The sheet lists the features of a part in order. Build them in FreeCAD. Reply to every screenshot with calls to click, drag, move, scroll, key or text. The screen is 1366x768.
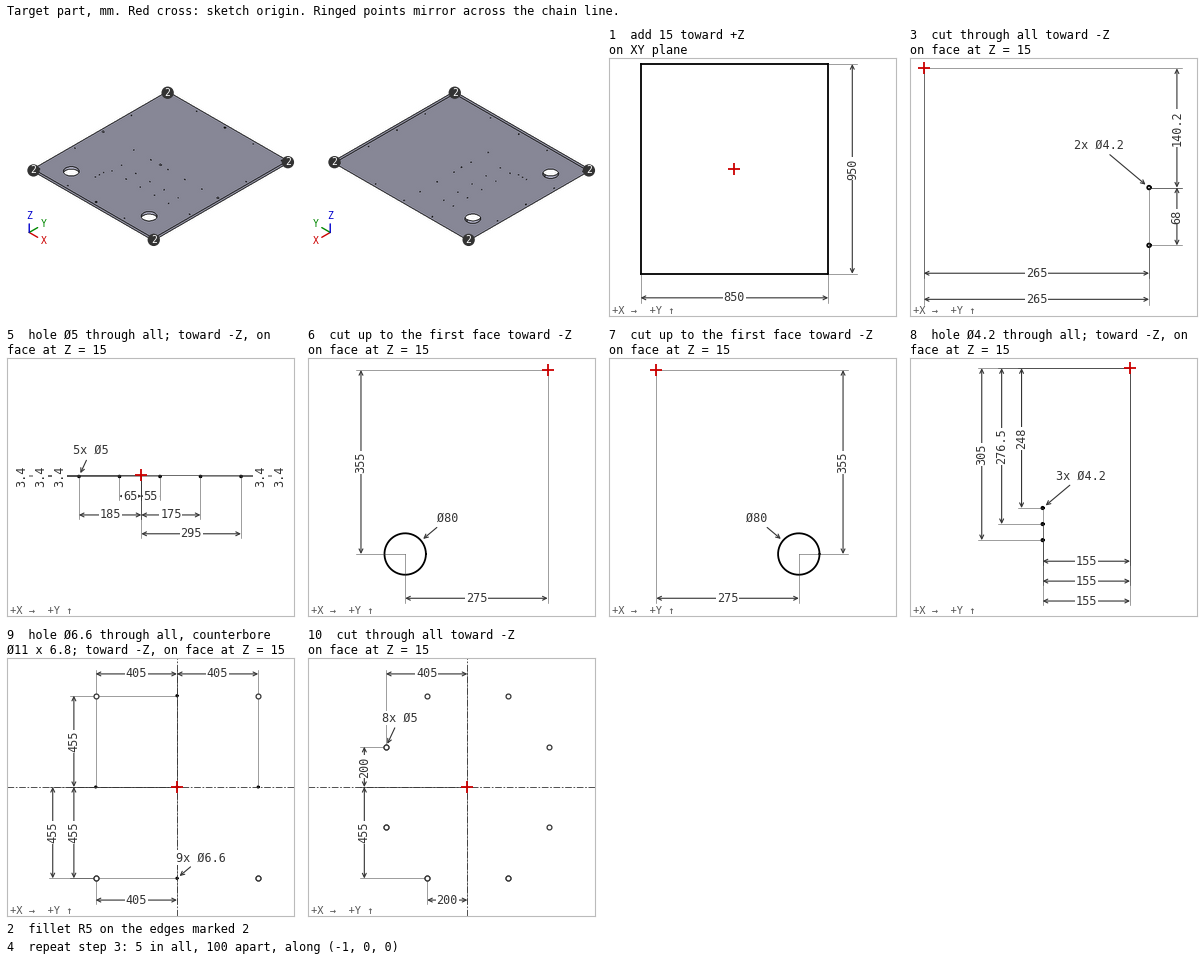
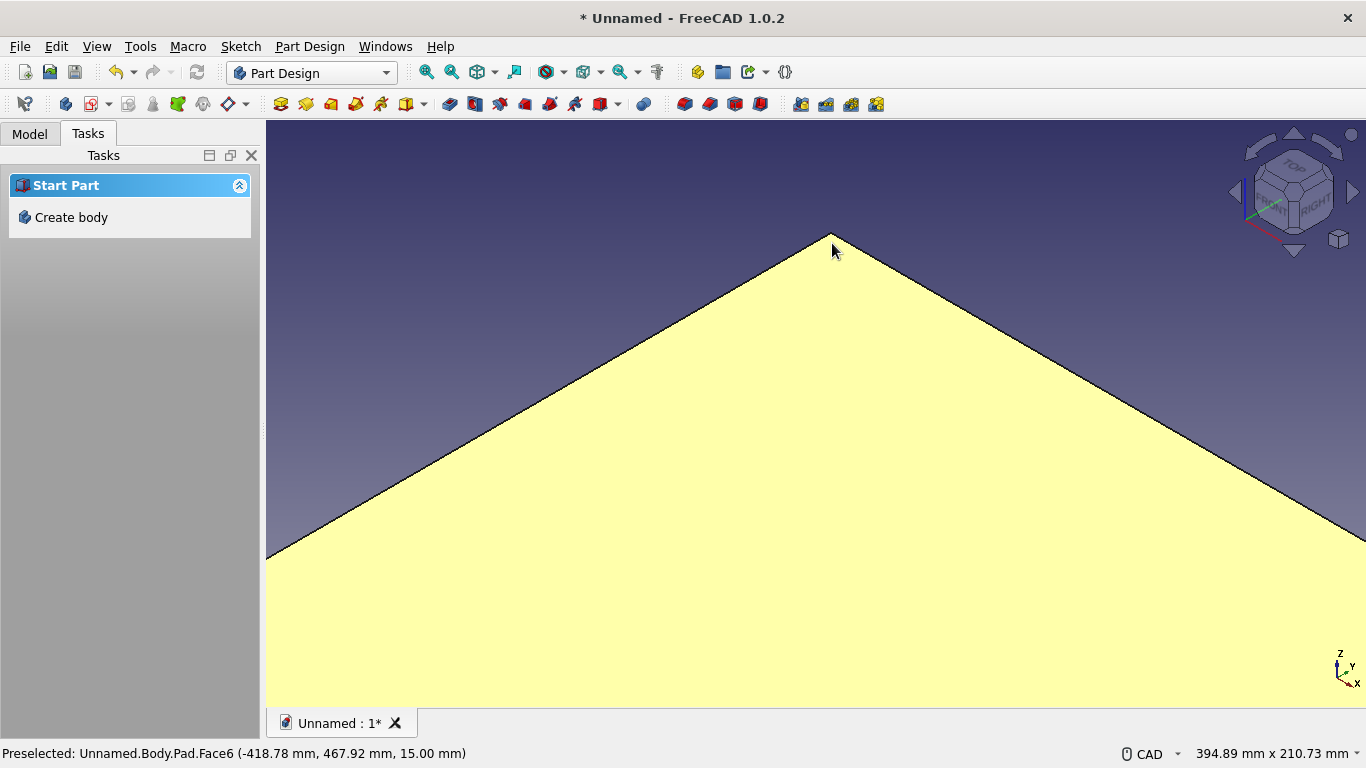
click(427, 72)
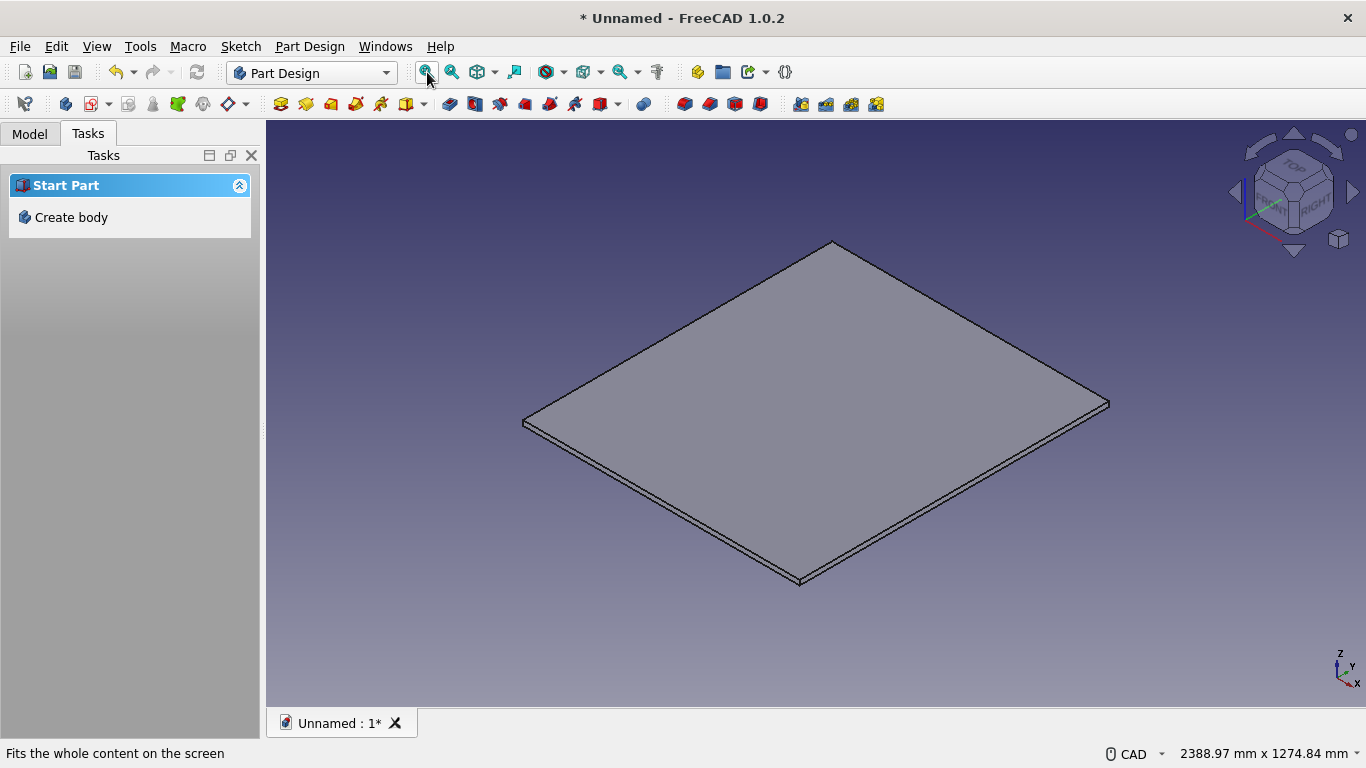
key(2)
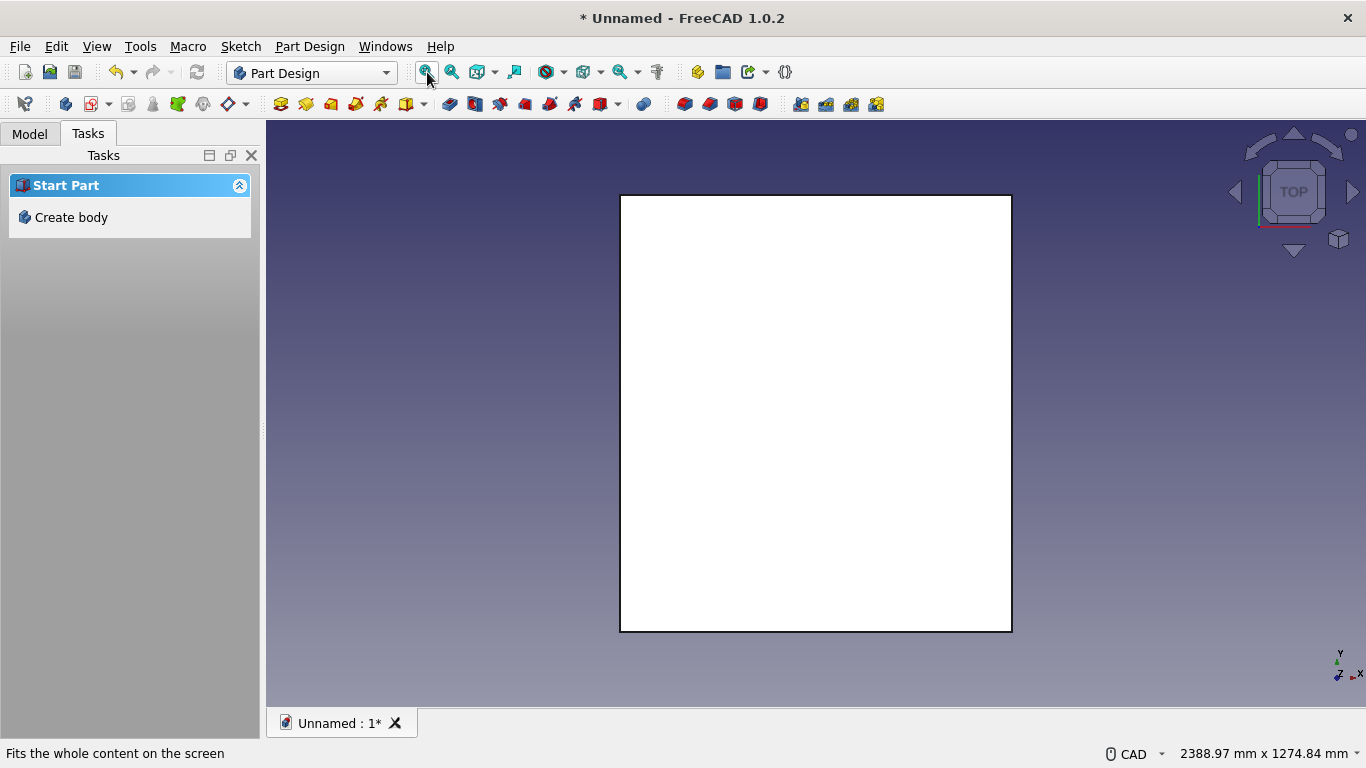
scroll(620, 194, up, 9)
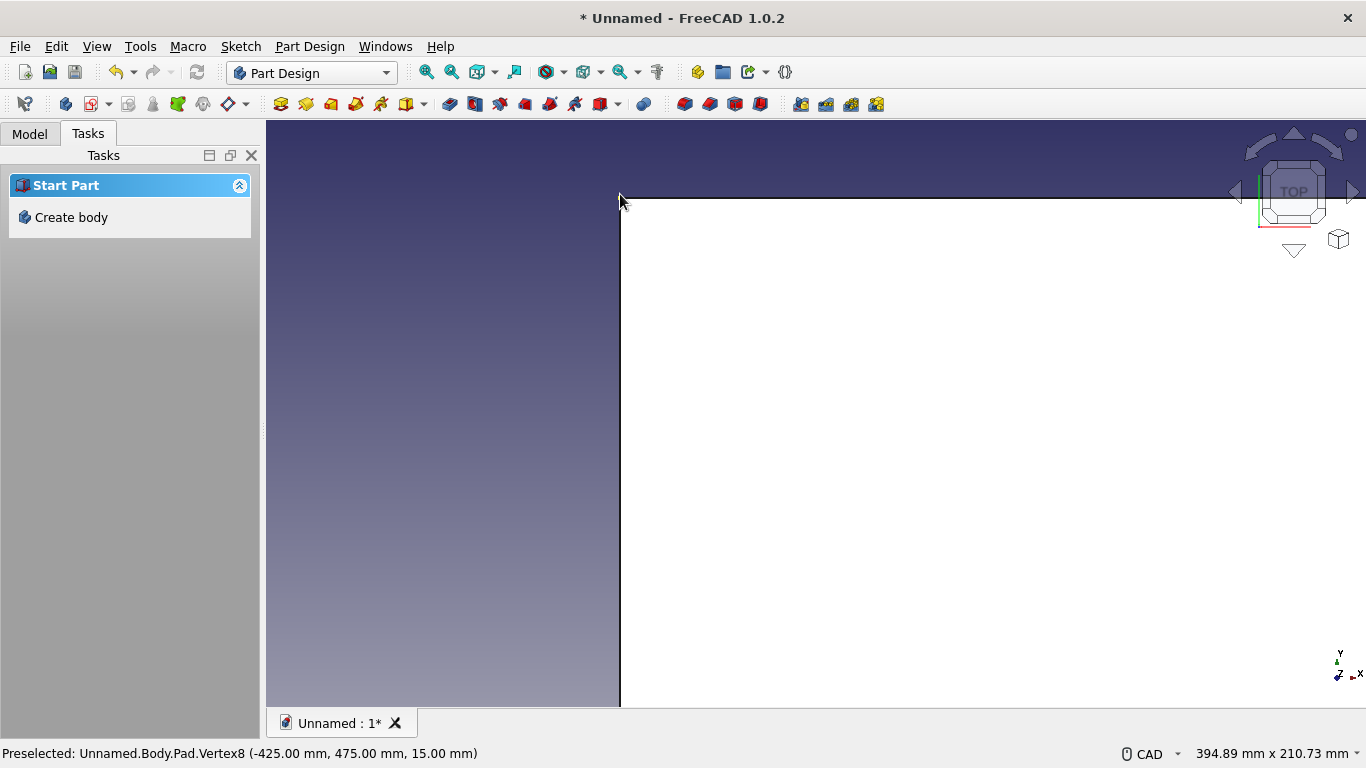
click(427, 72)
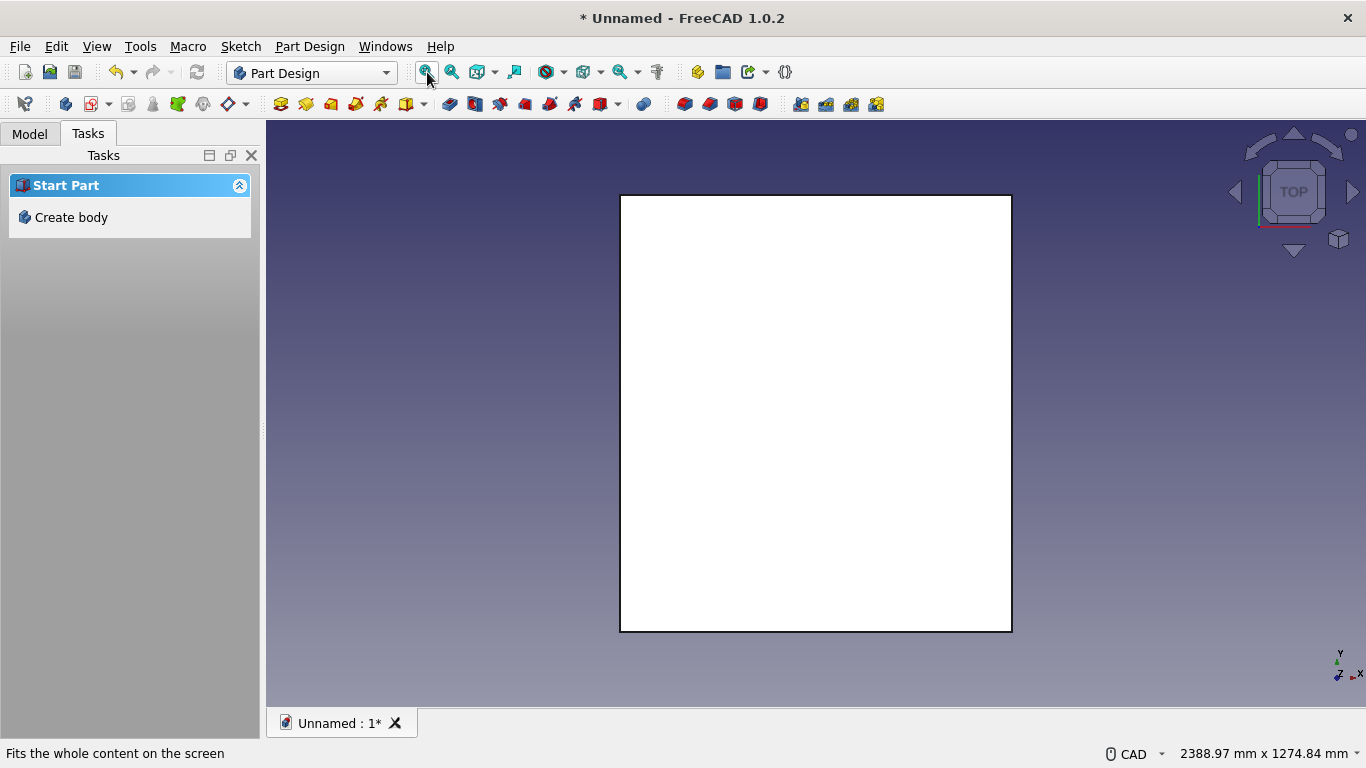
key(1)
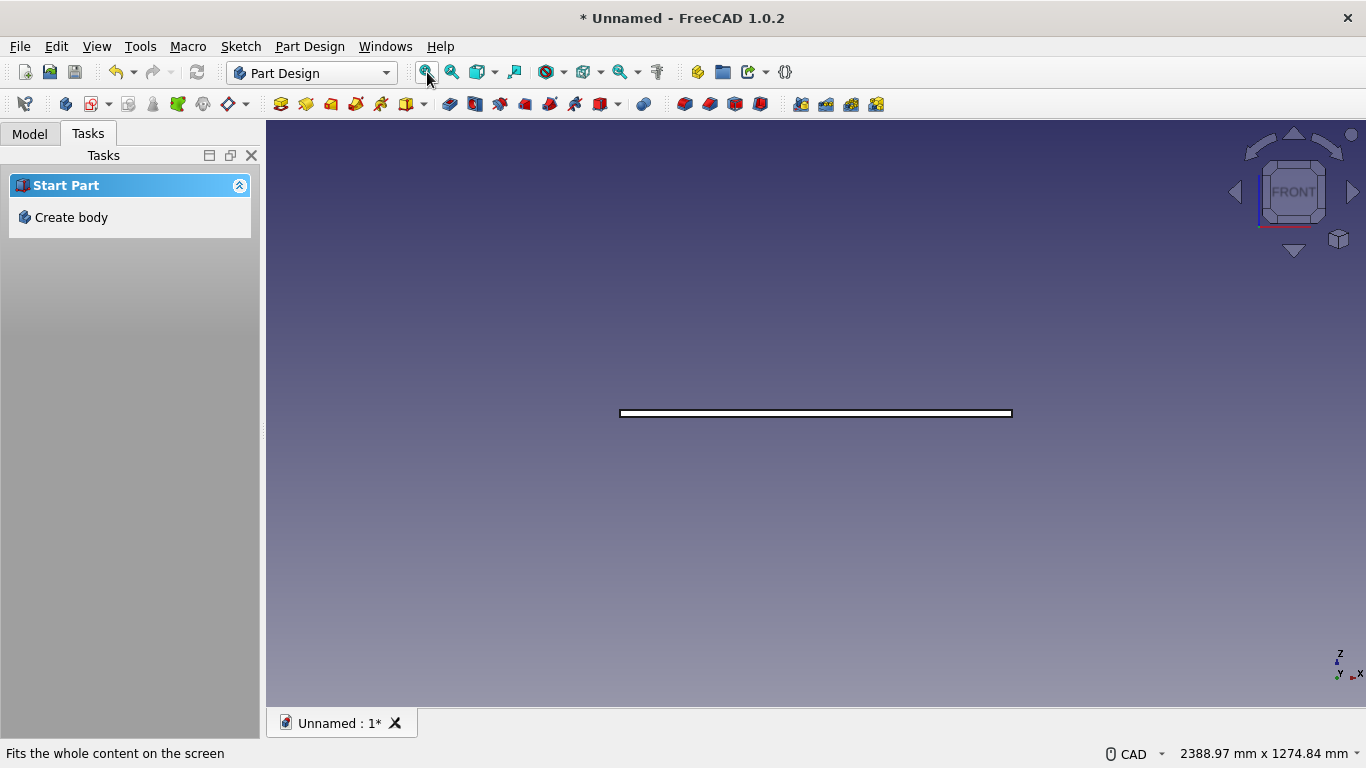
click(427, 72)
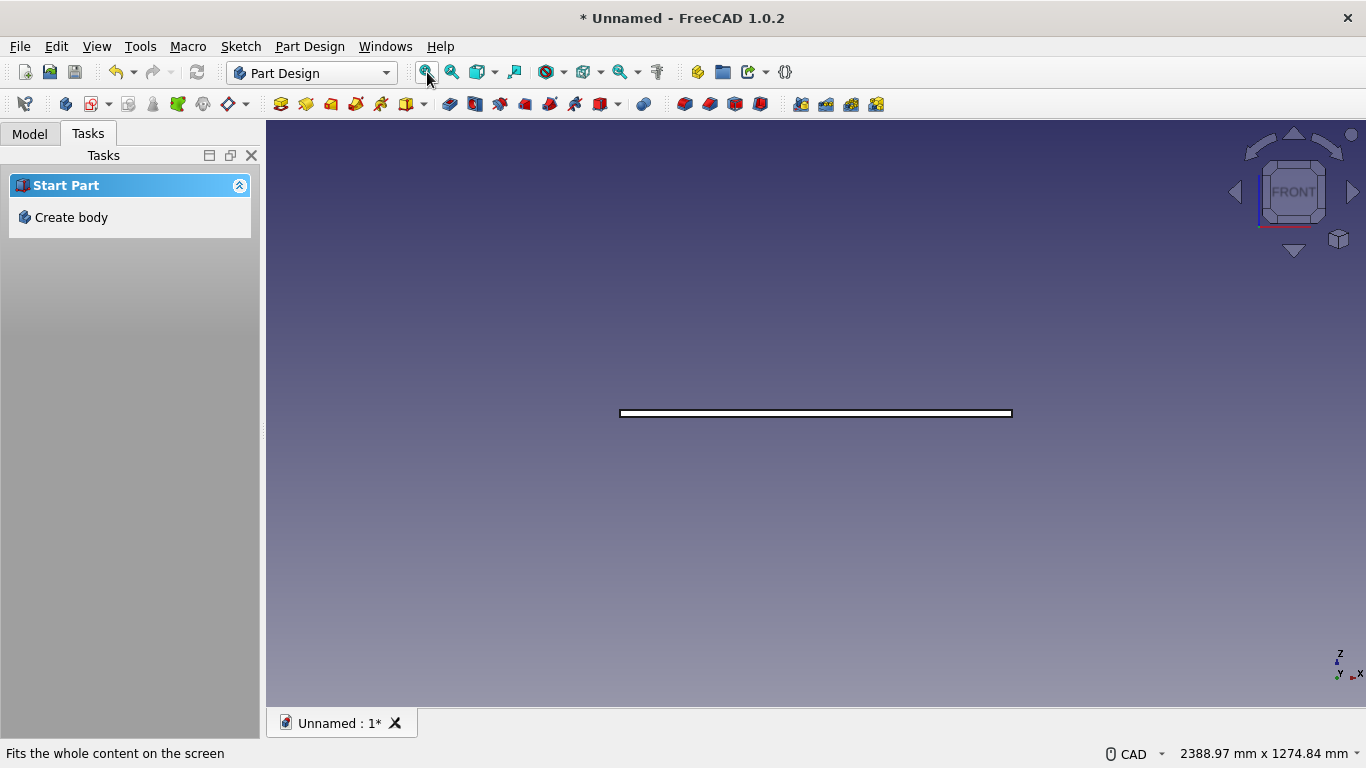
scroll(620, 413, up, 9)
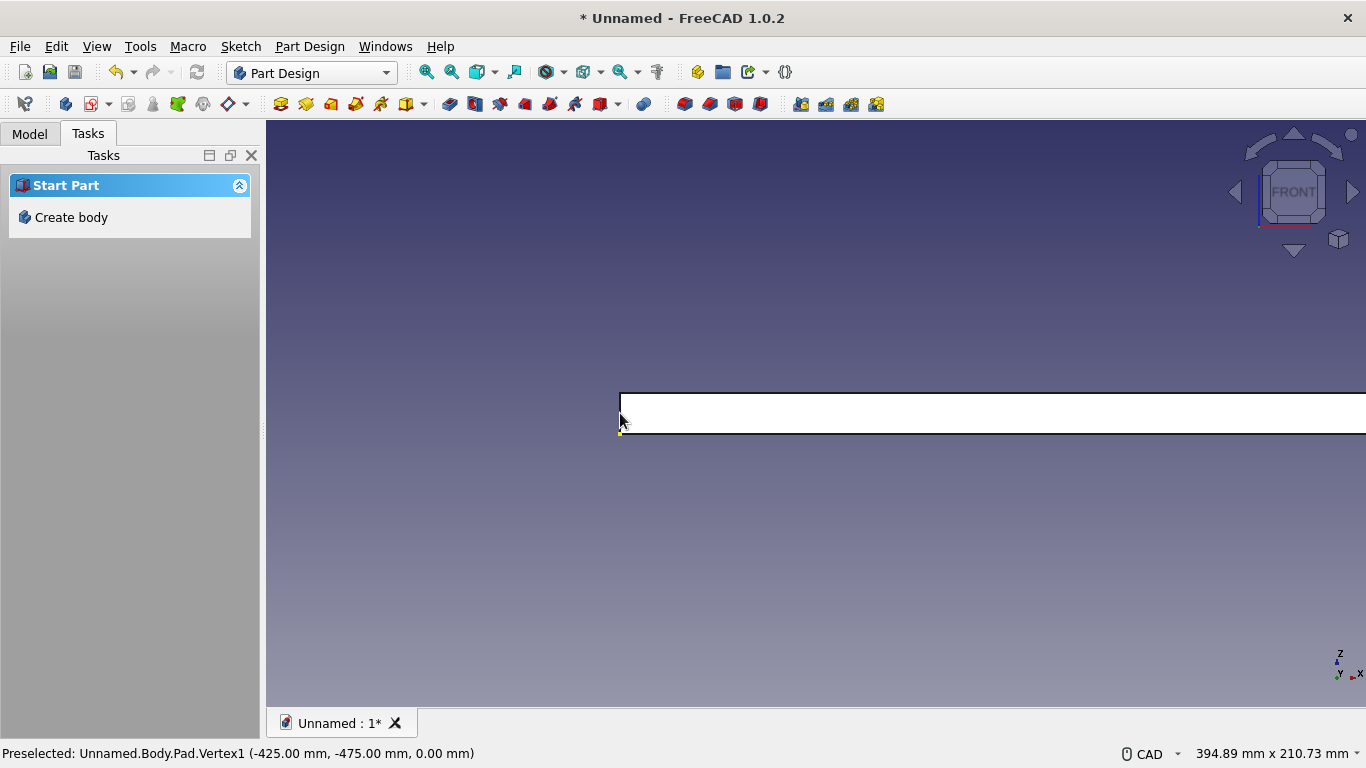
click(620, 413)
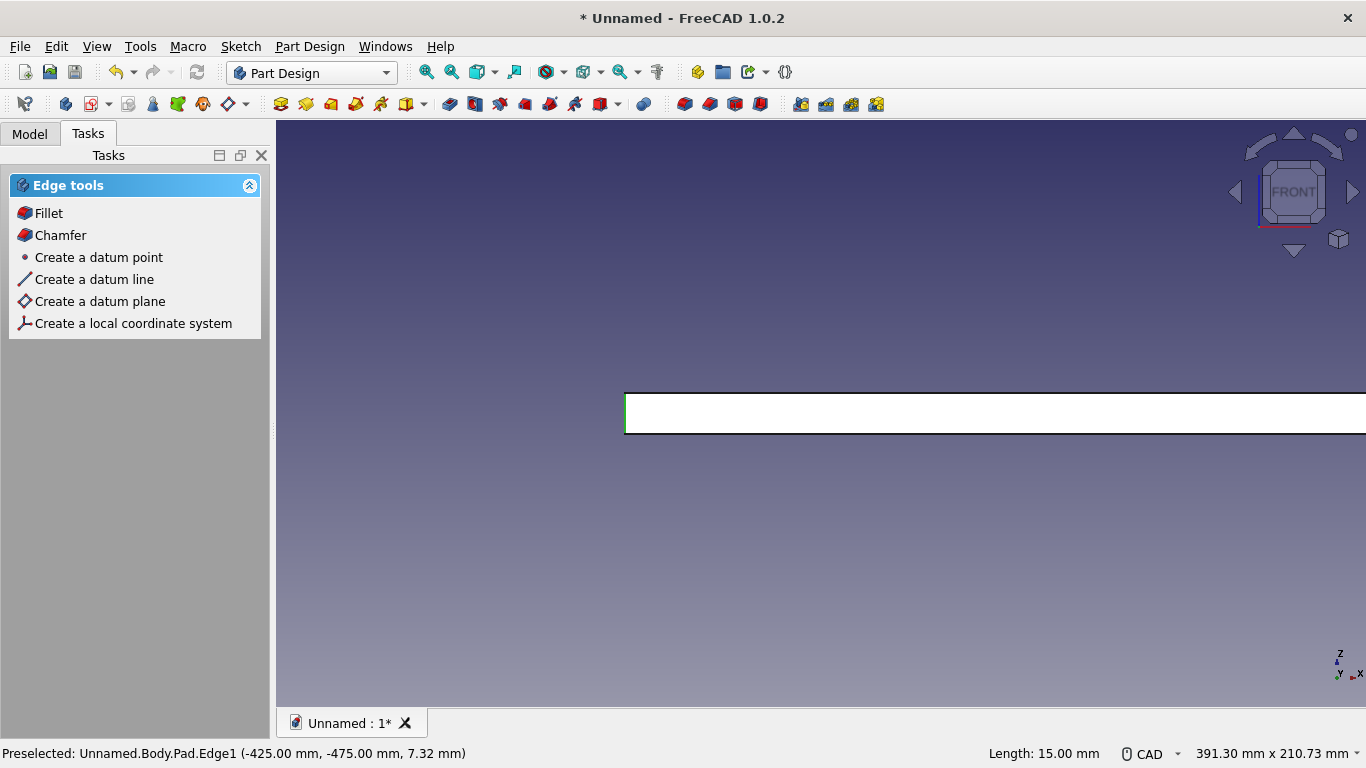
click(427, 72)